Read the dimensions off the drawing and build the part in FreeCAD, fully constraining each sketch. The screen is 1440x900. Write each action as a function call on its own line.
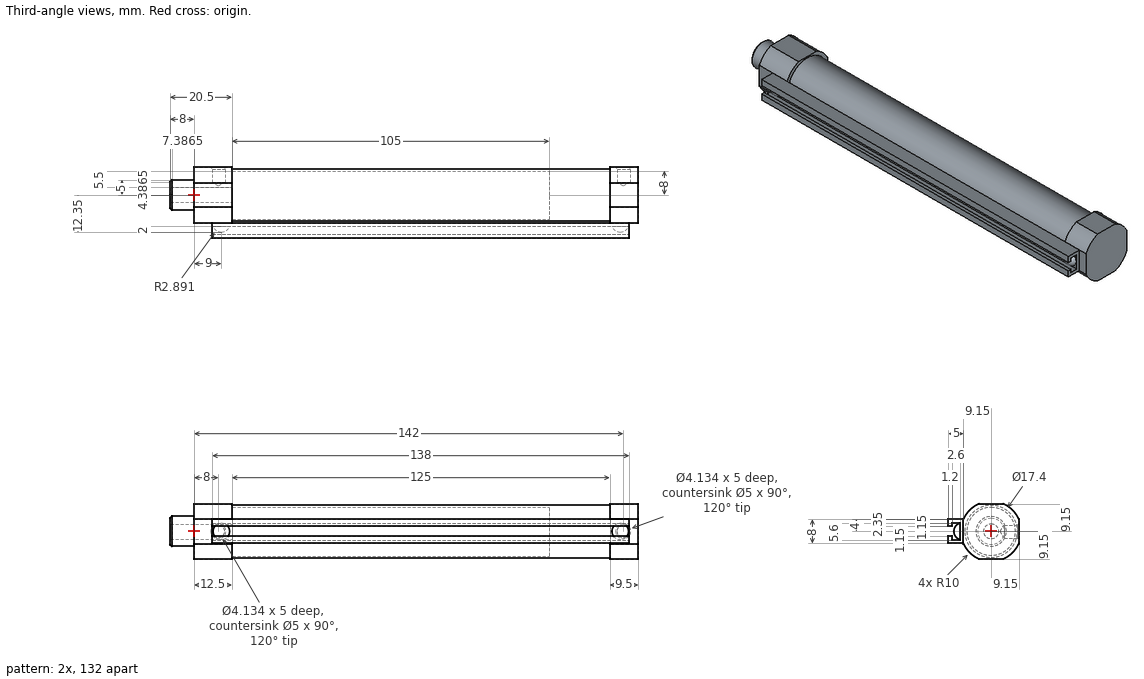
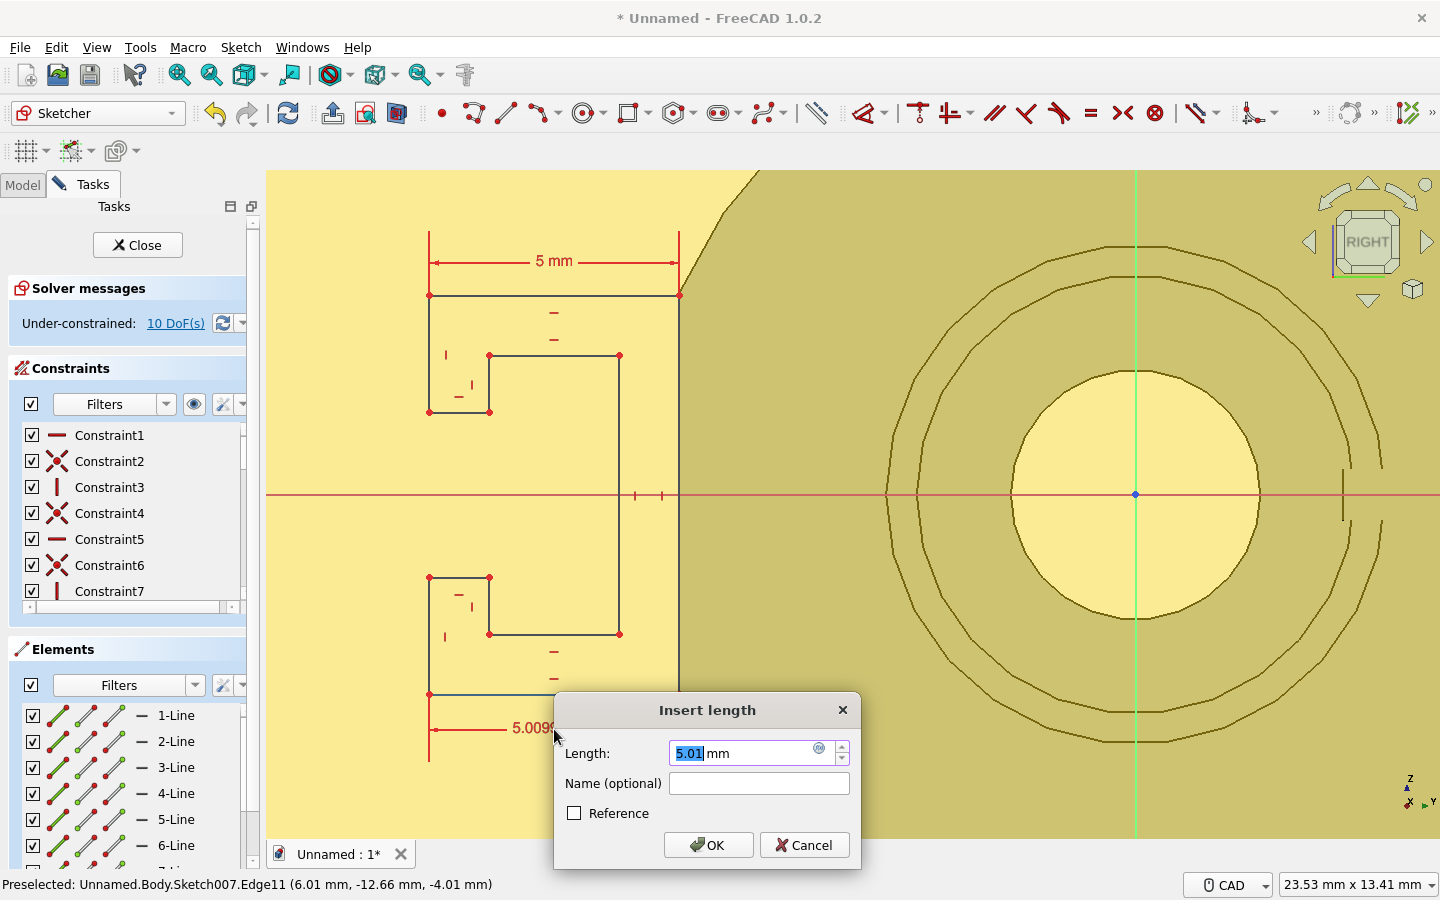
text(5)
key(Return)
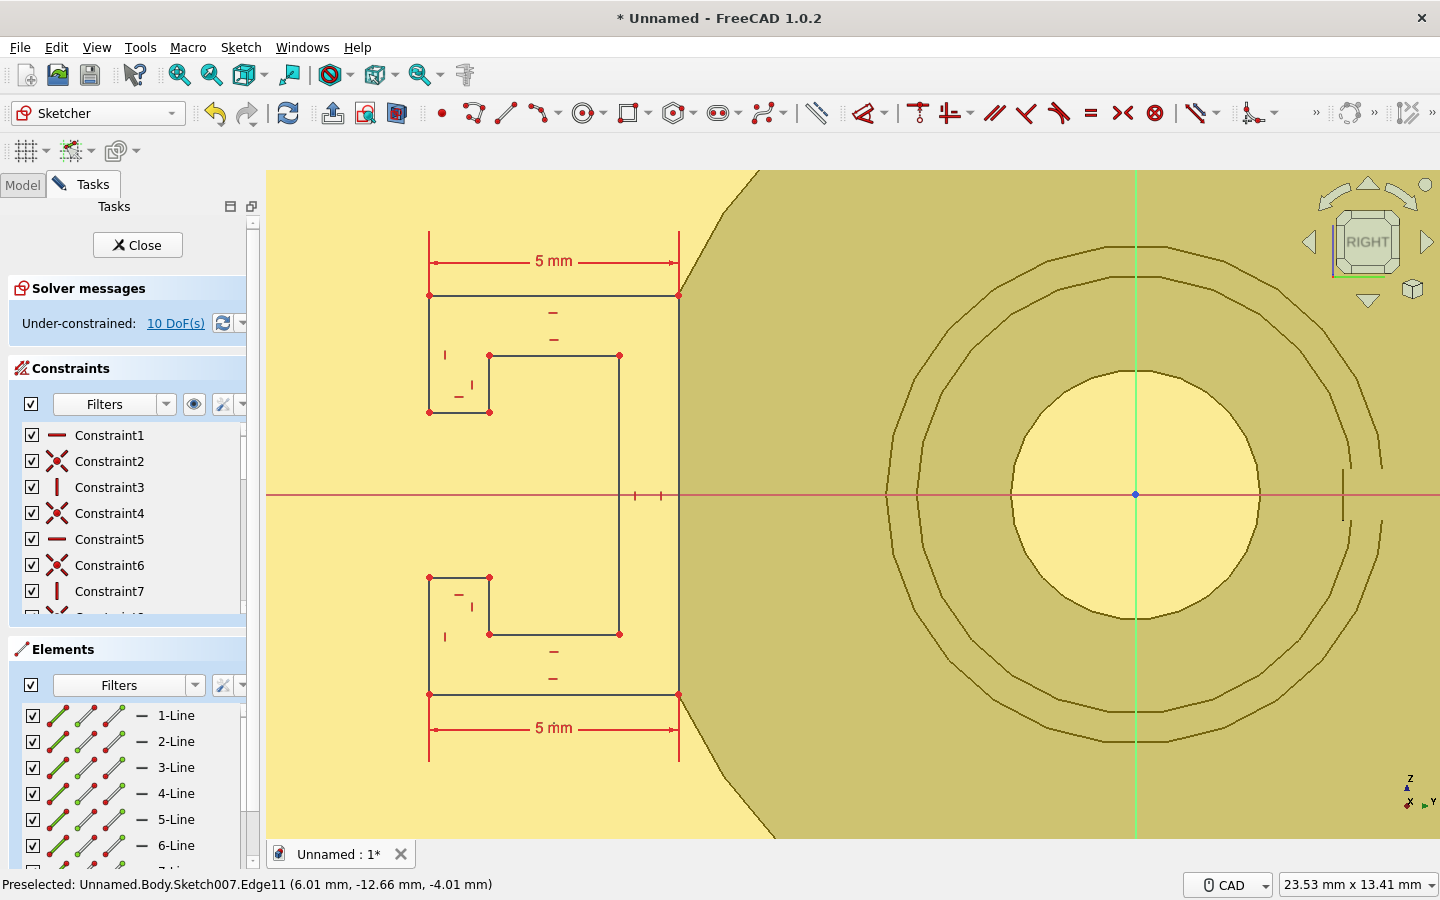
click(679, 575)
click(645, 404)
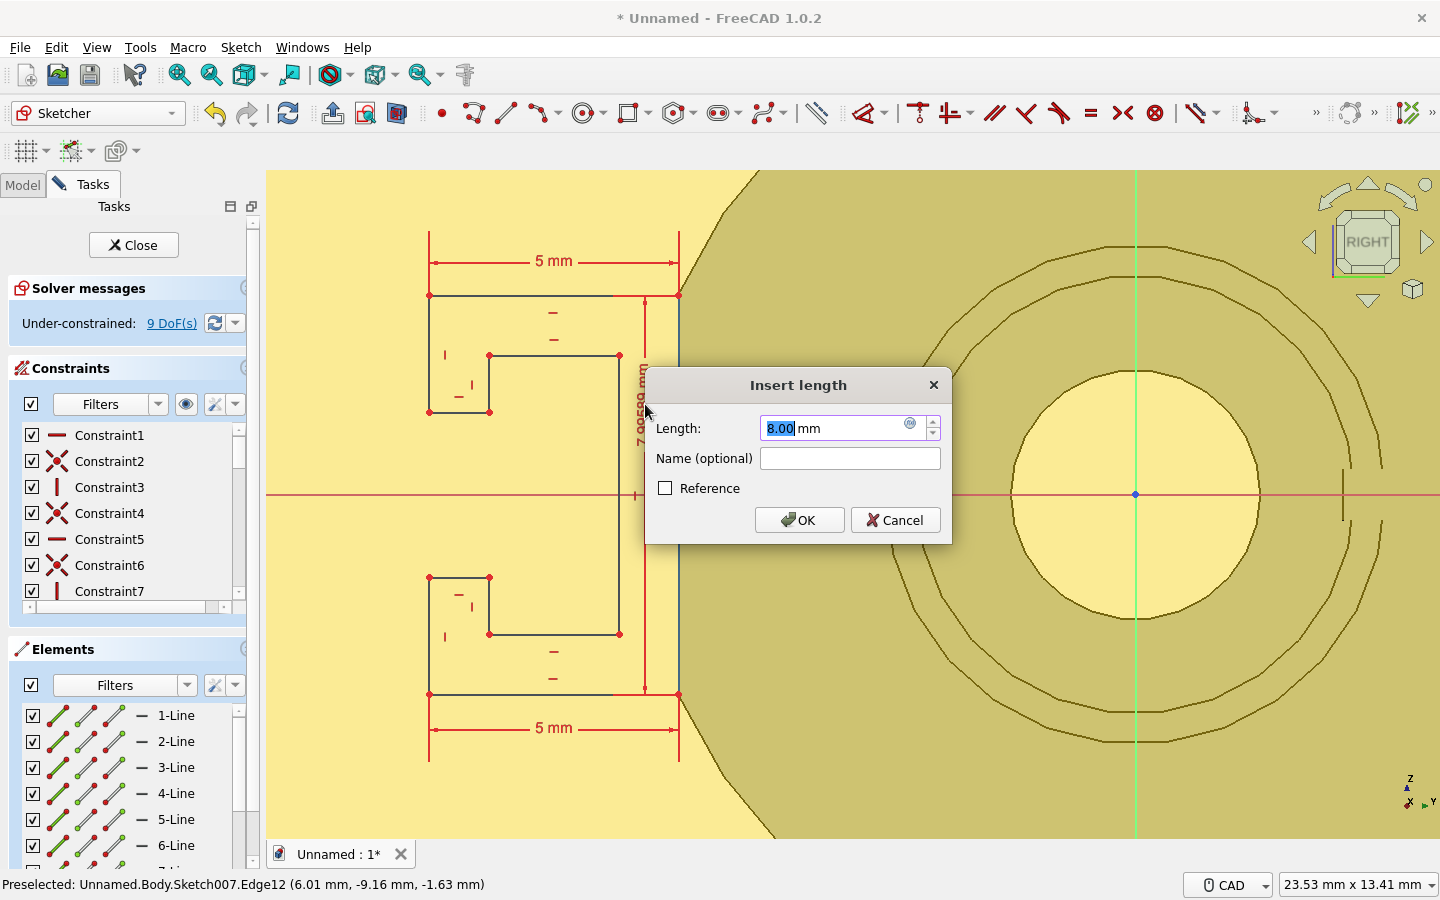
text(8)
key(Return)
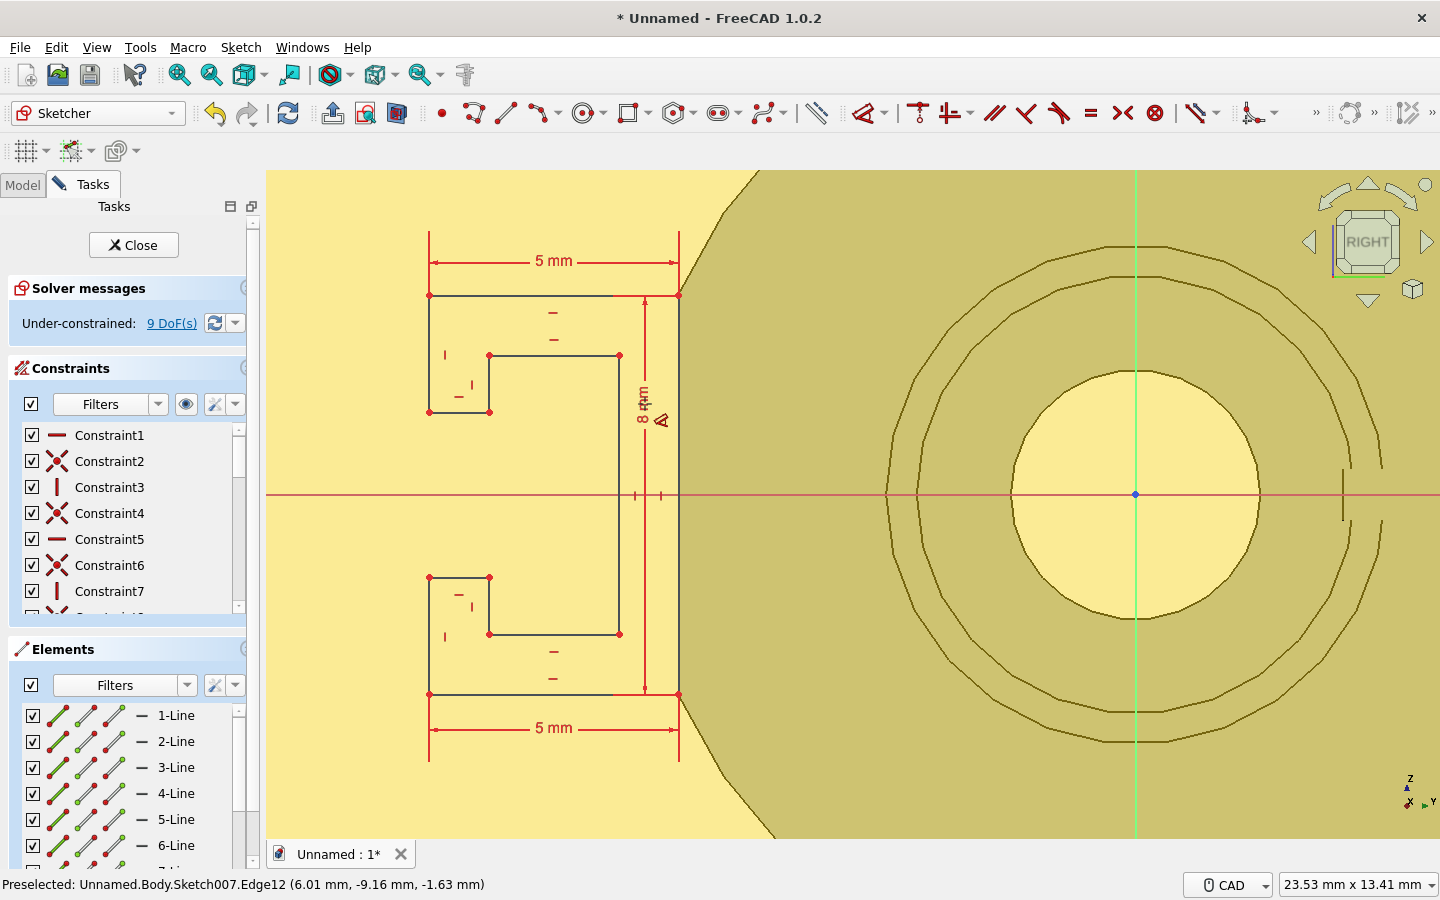
click(679, 296)
click(1170, 395)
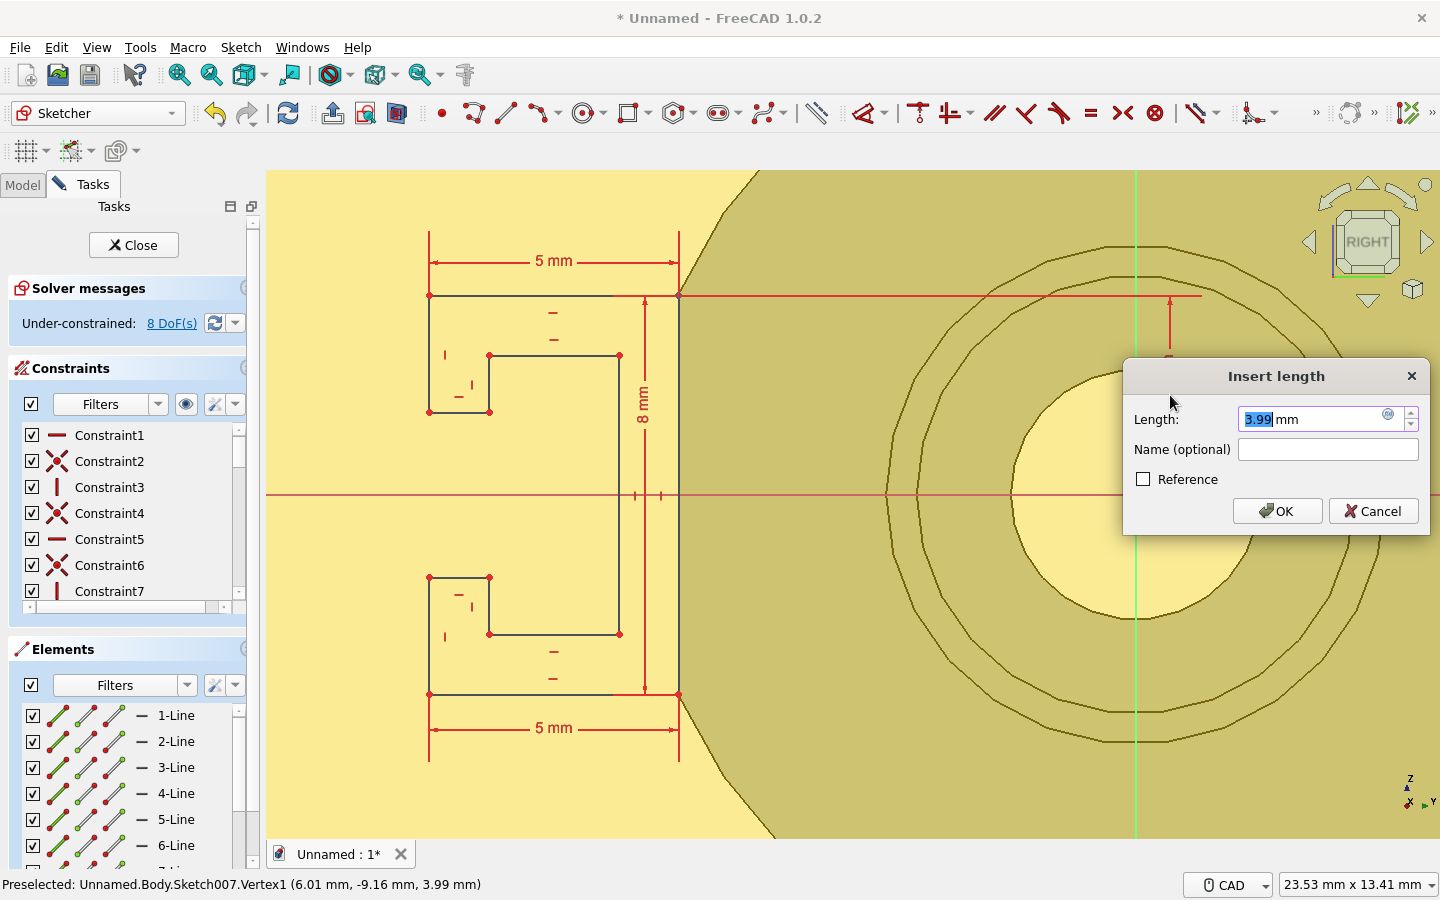
text(4)
key(Return)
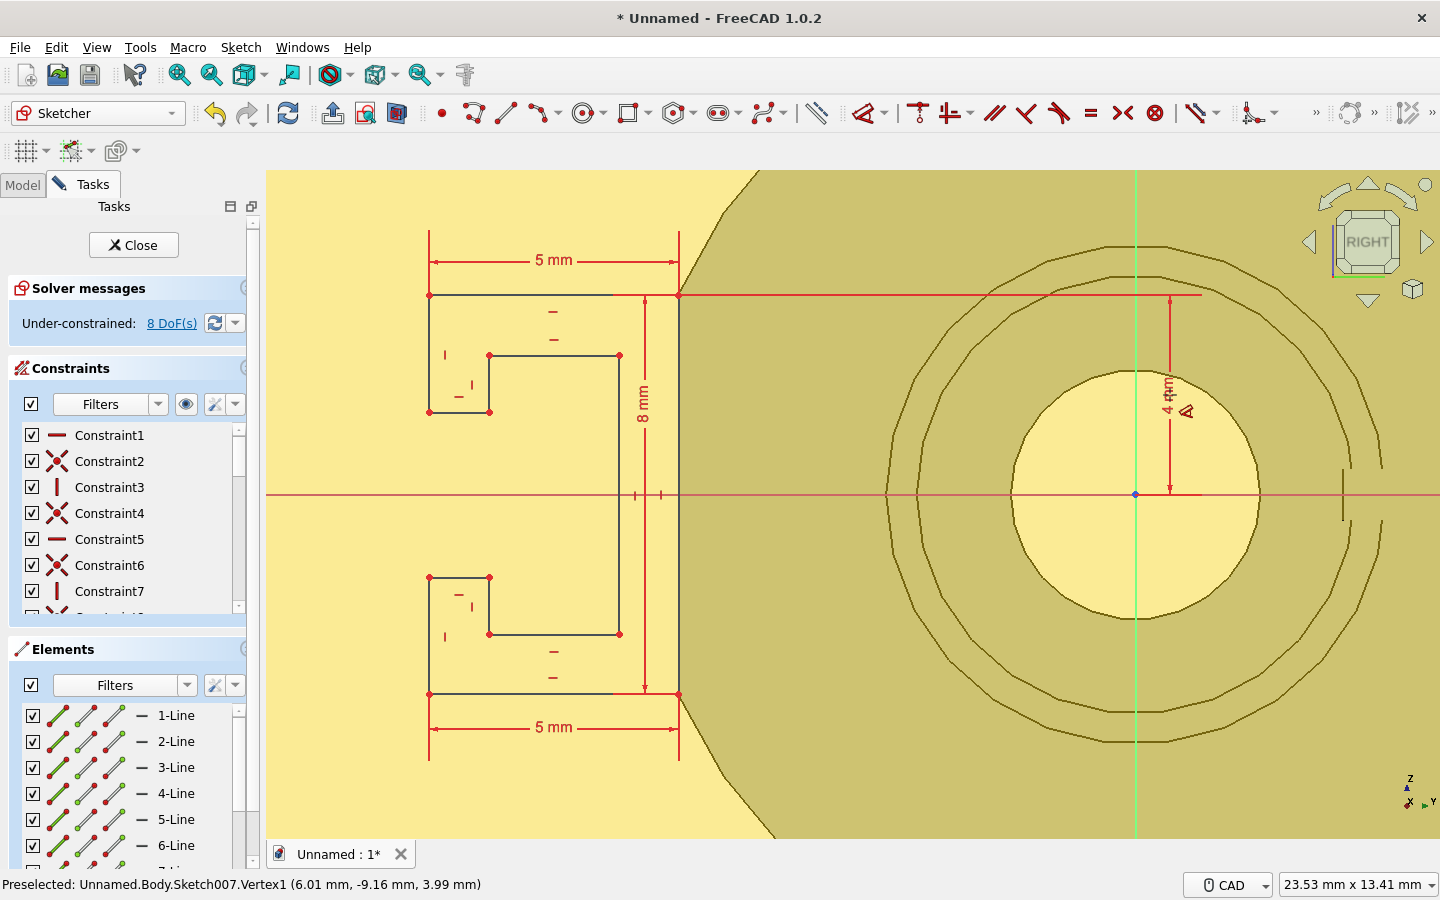
click(447, 413)
click(459, 379)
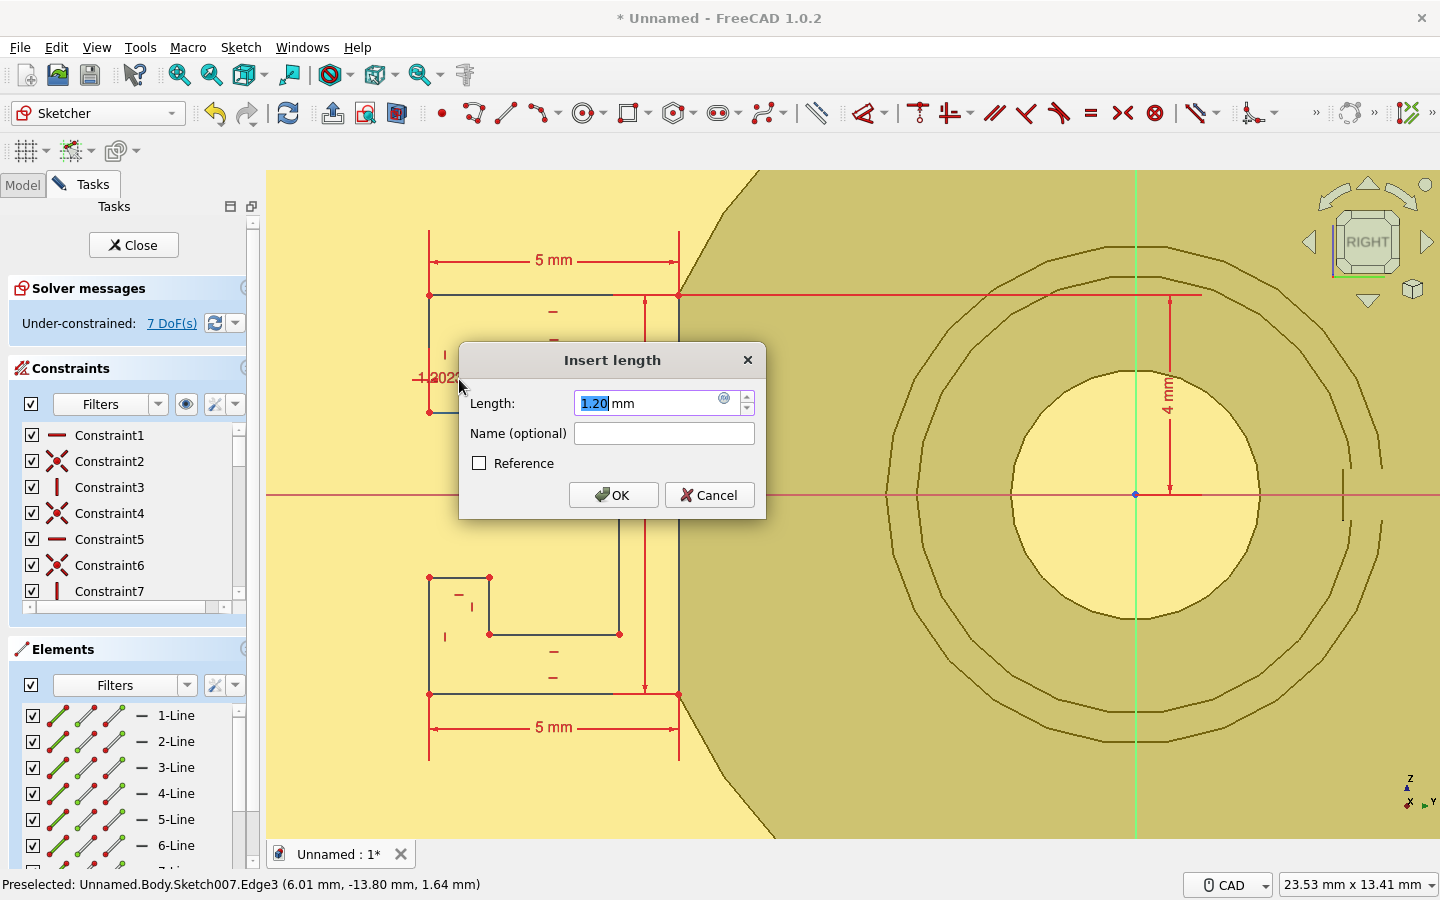
text(1.2)
key(Return)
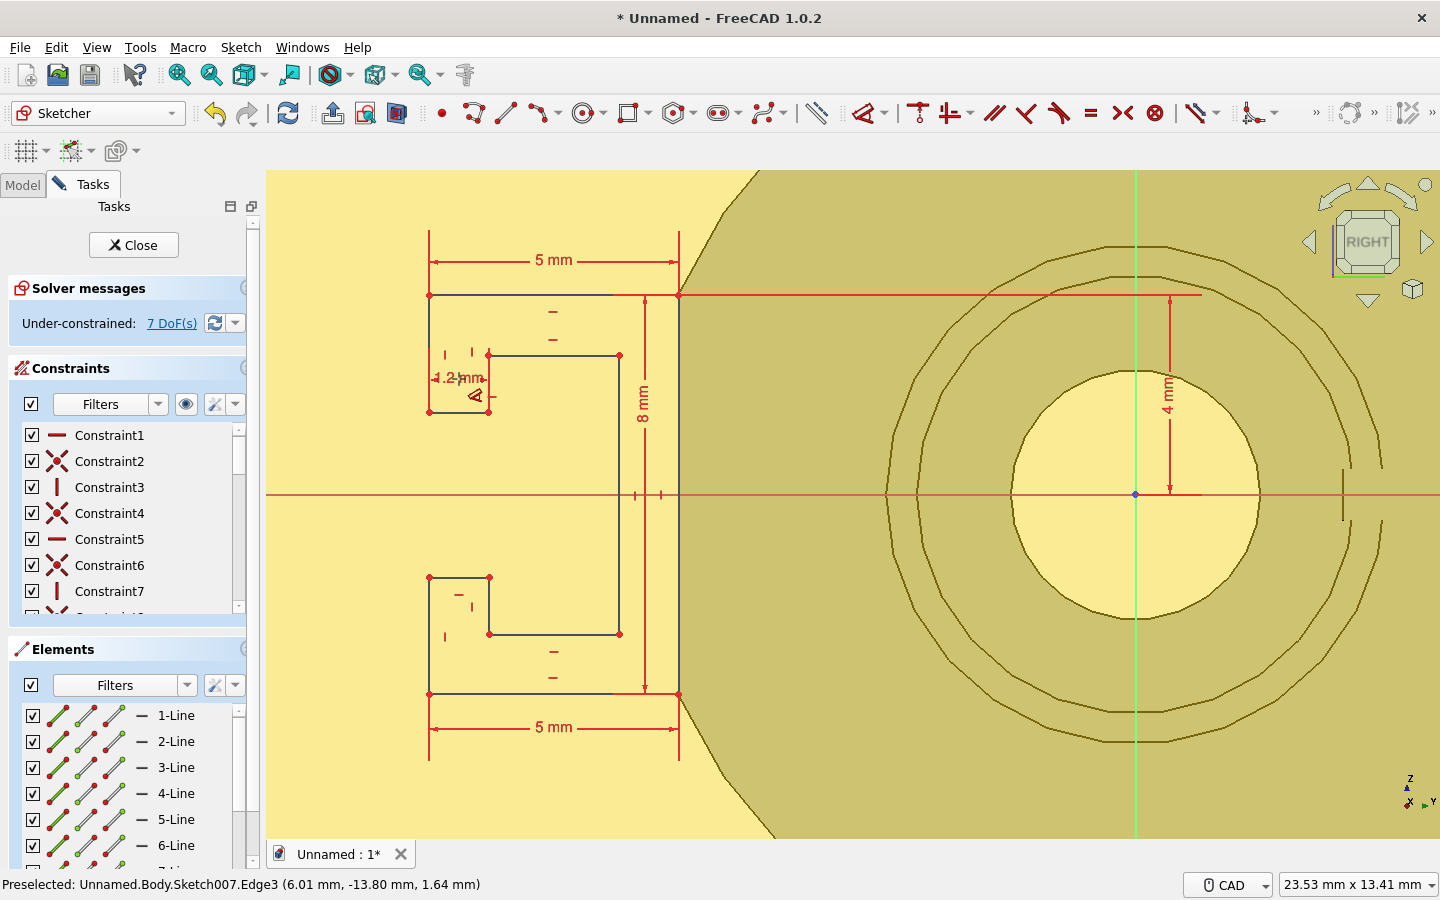
click(528, 356)
click(554, 322)